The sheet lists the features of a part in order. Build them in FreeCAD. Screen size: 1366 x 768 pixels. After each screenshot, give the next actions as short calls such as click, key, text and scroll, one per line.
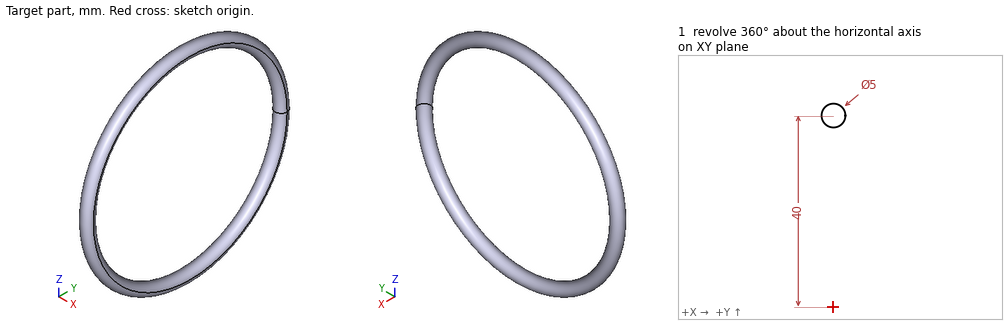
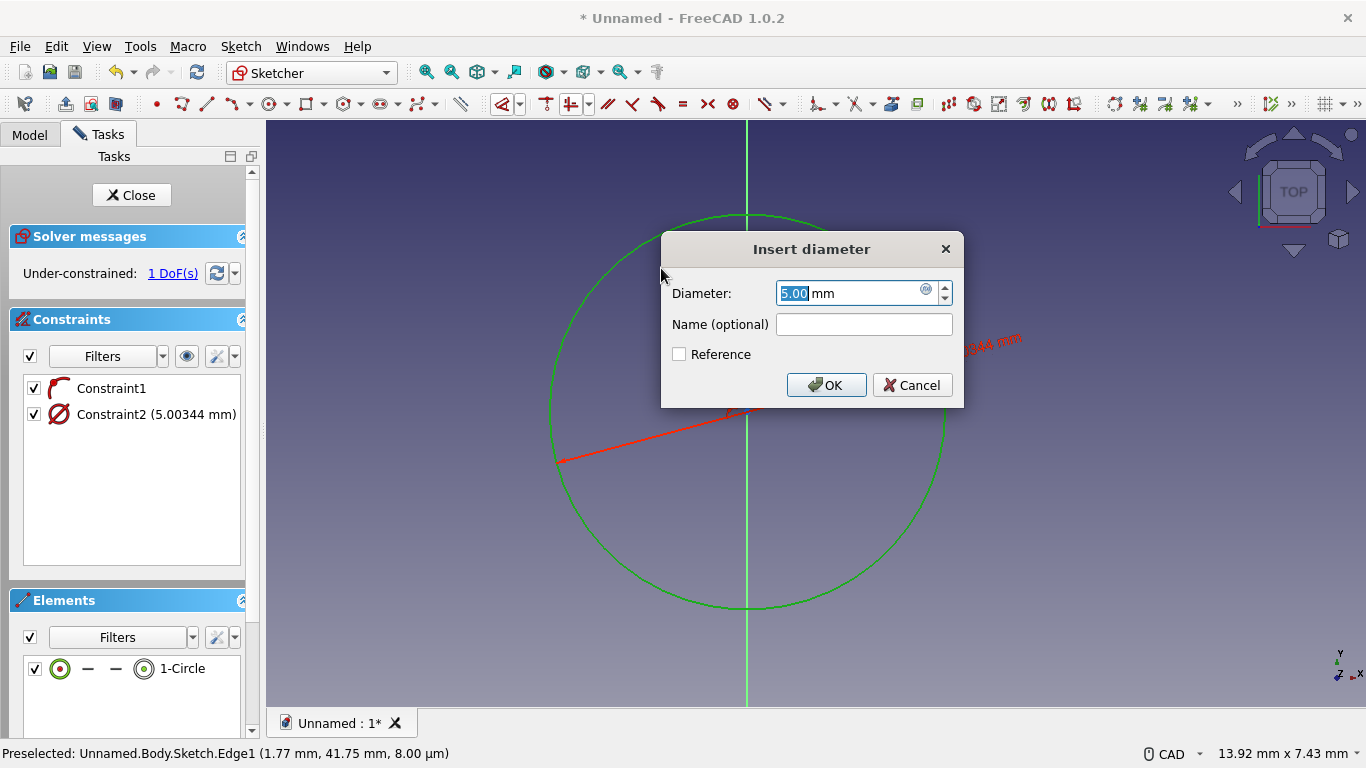
text(5)
key(Return)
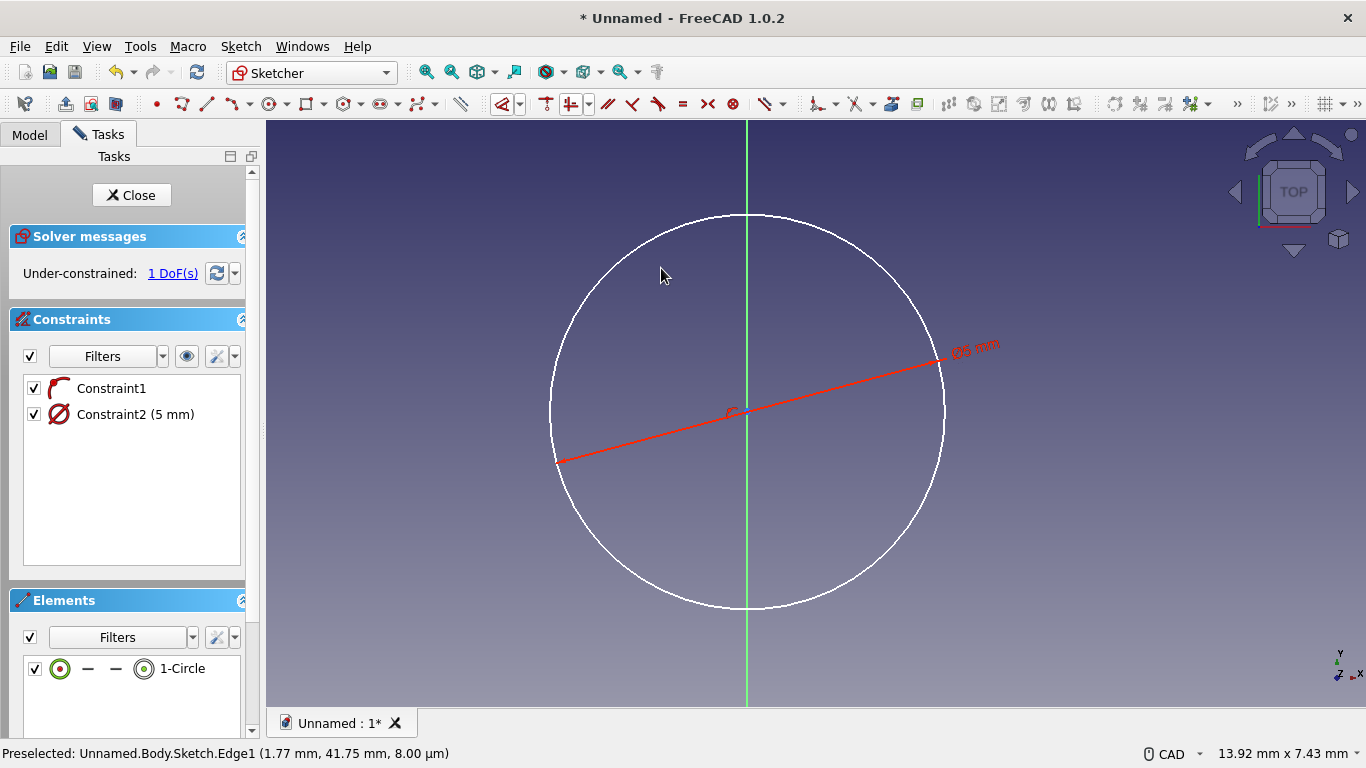
click(747, 412)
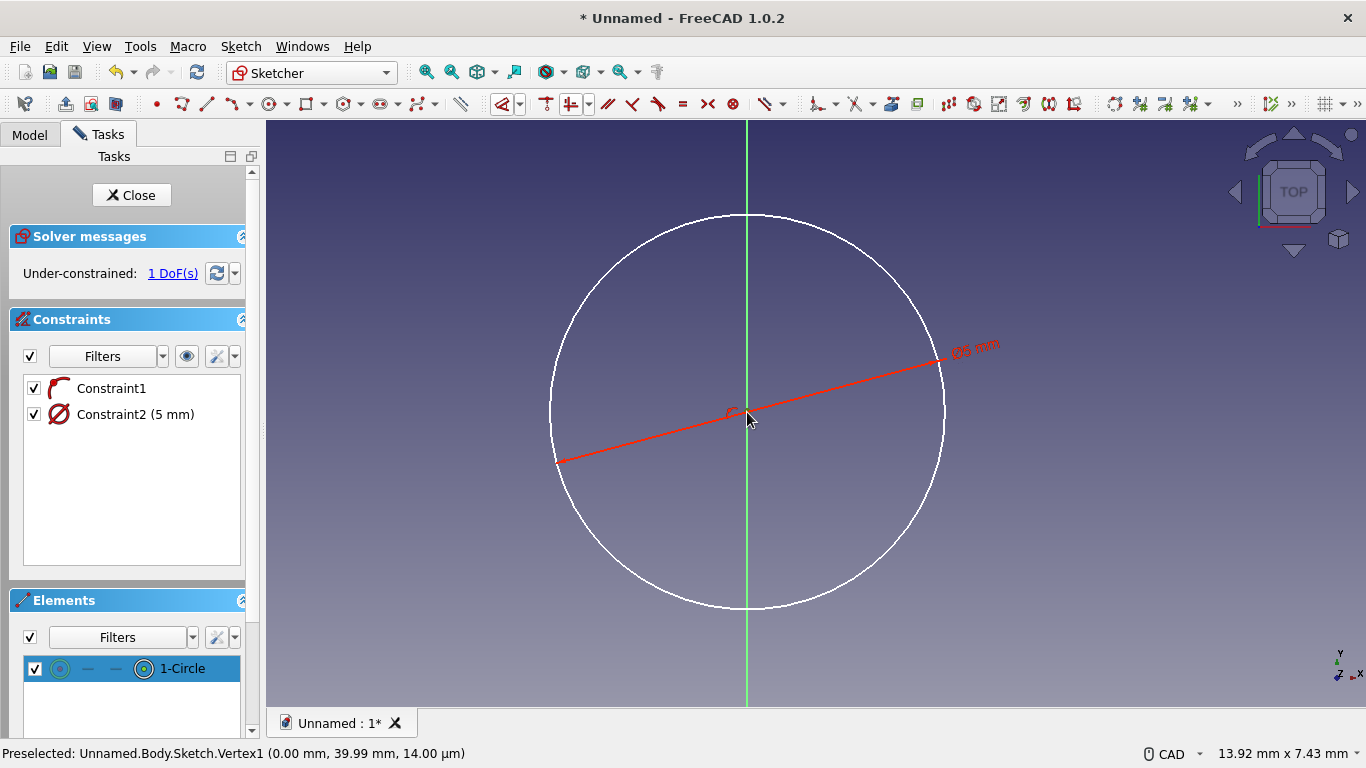
click(520, 104)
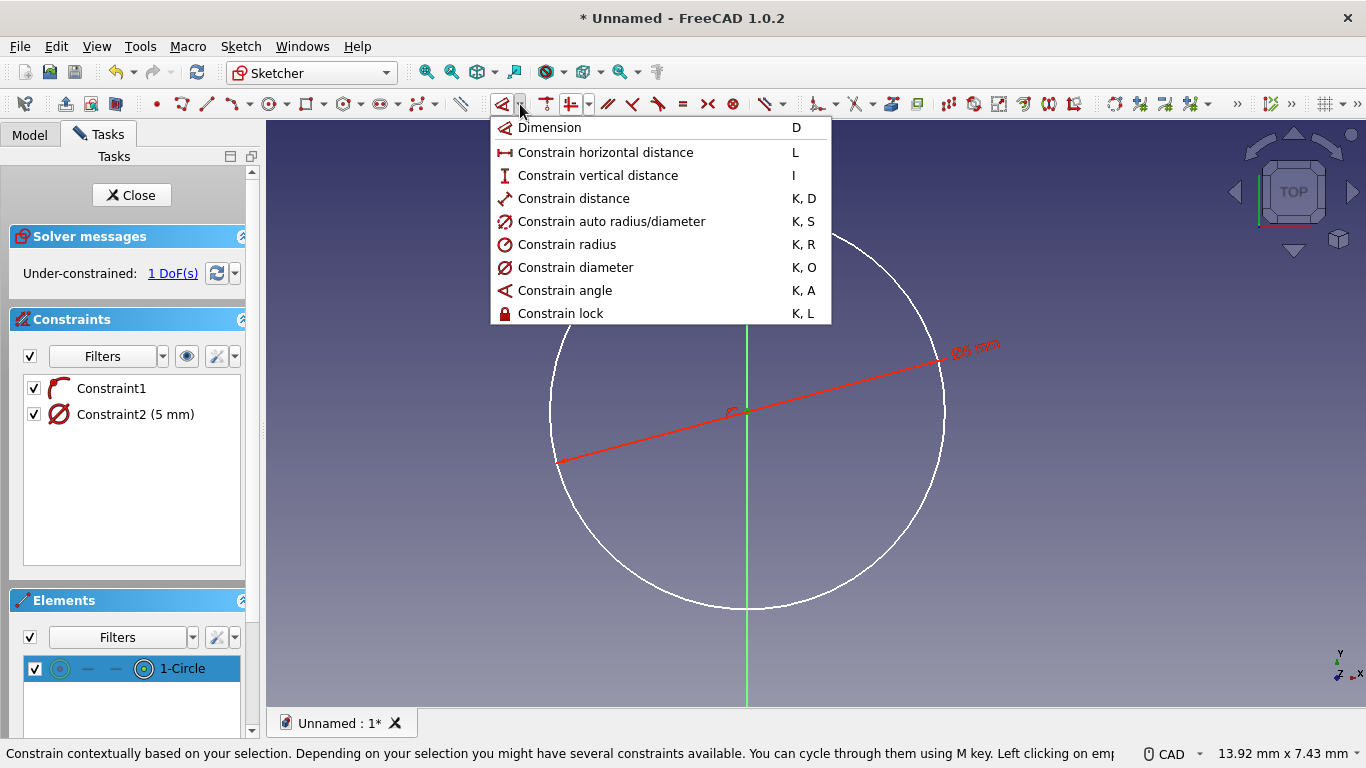
click(661, 176)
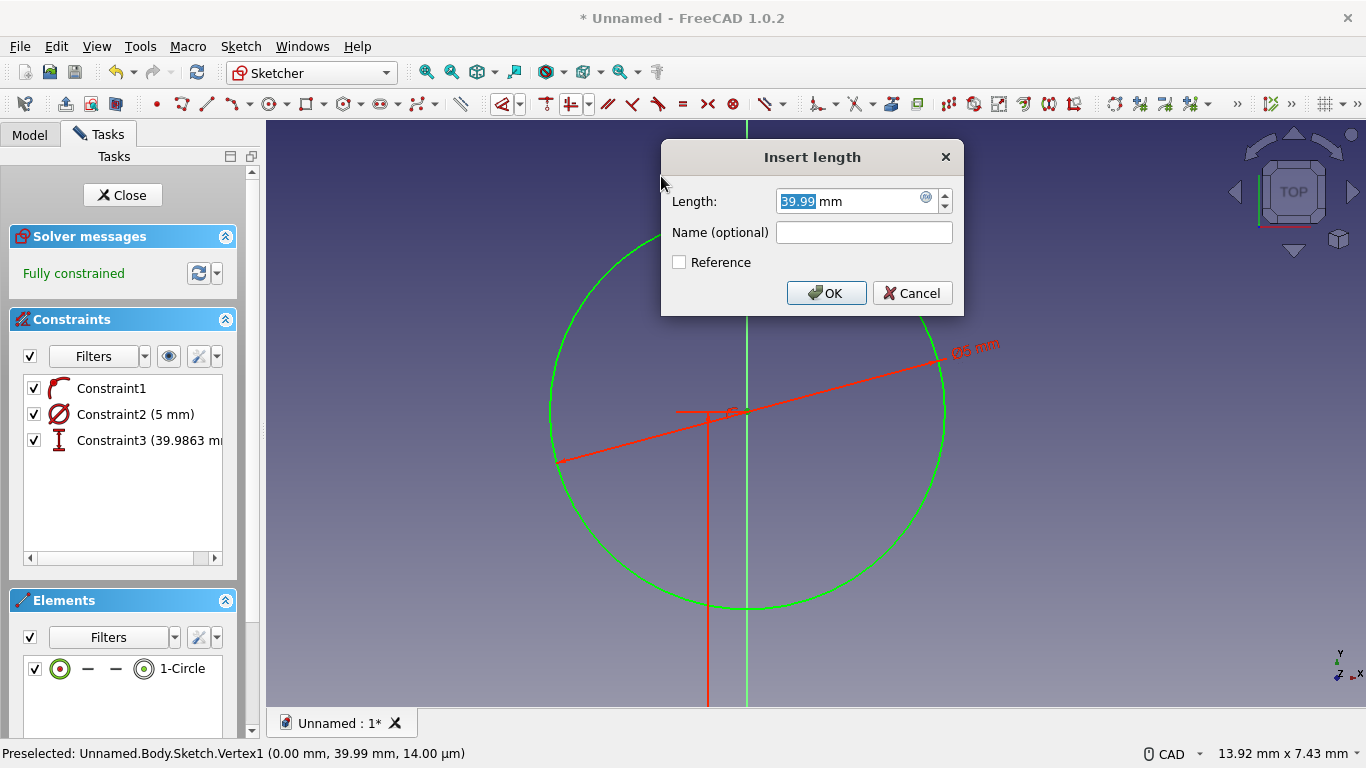
text(40)
key(Return)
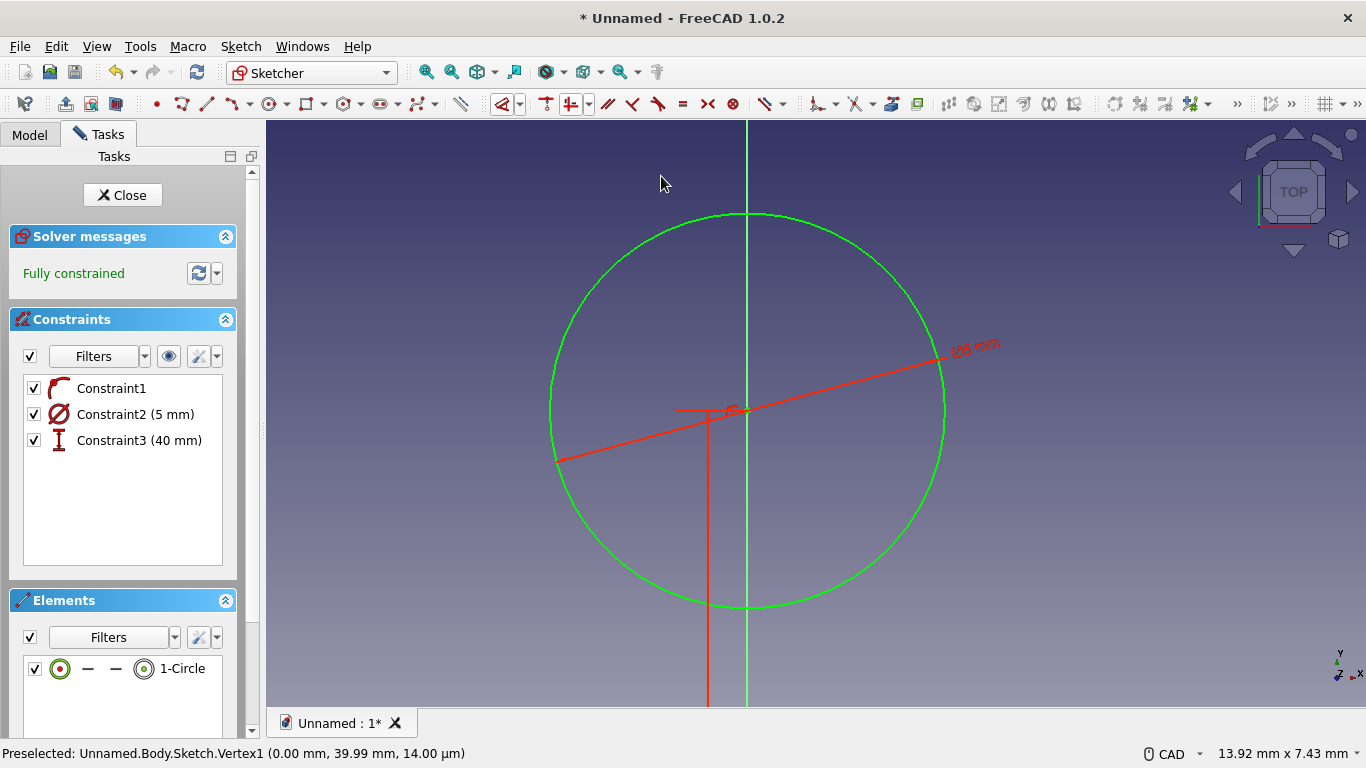
click(123, 195)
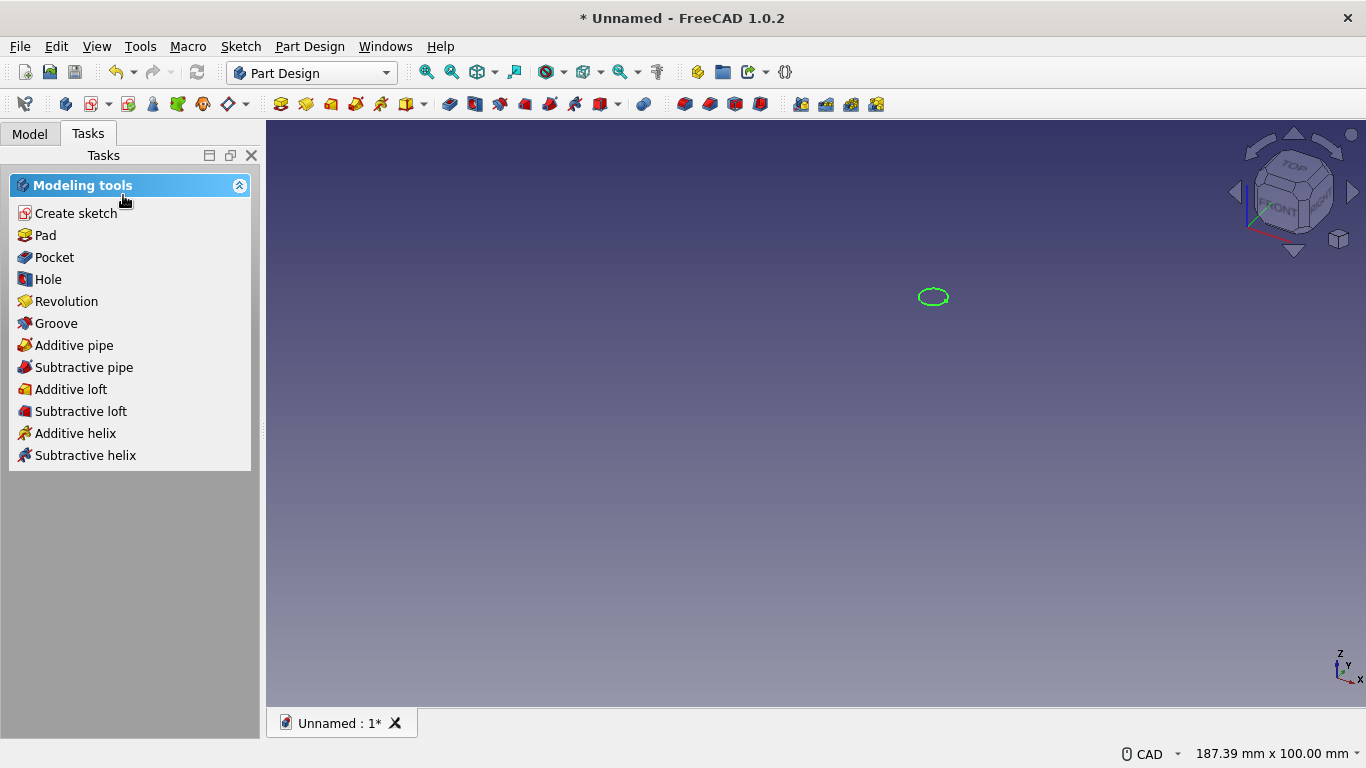
click(306, 104)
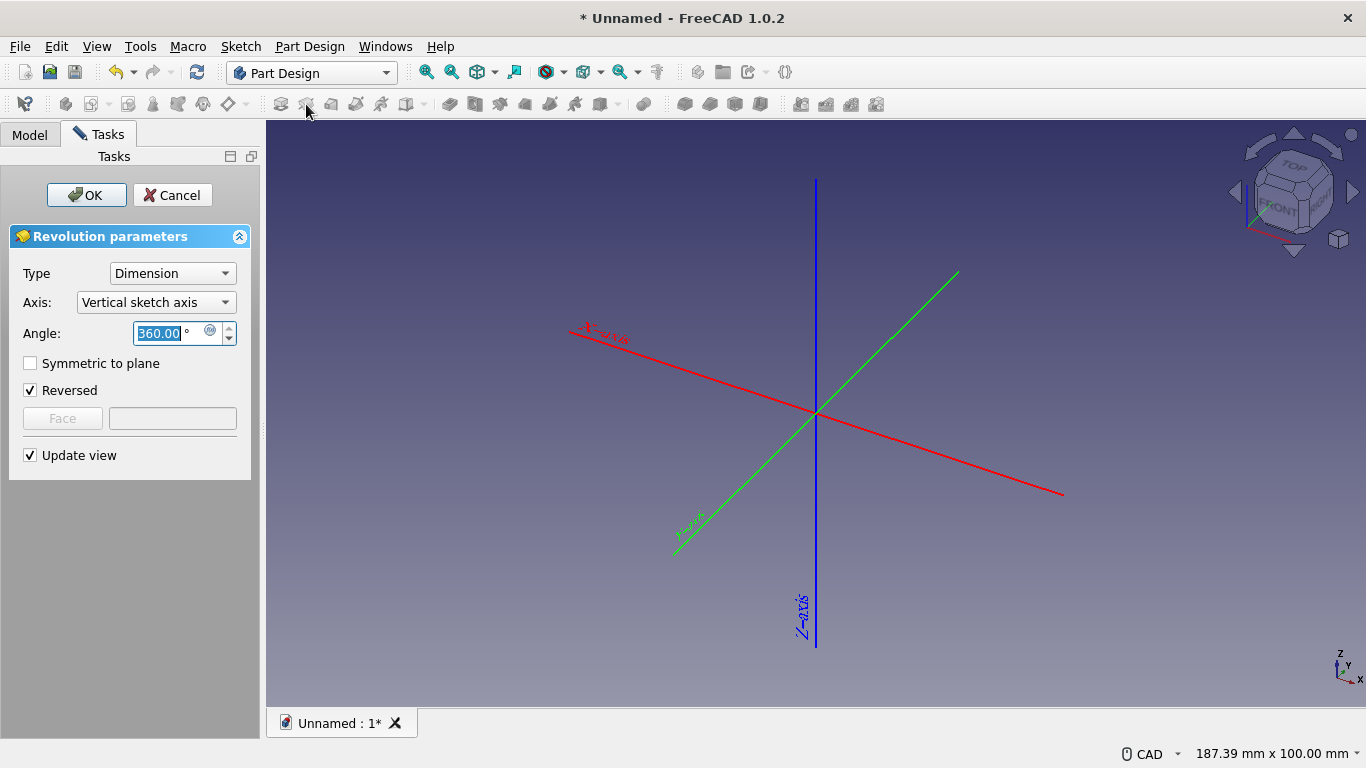
click(157, 302)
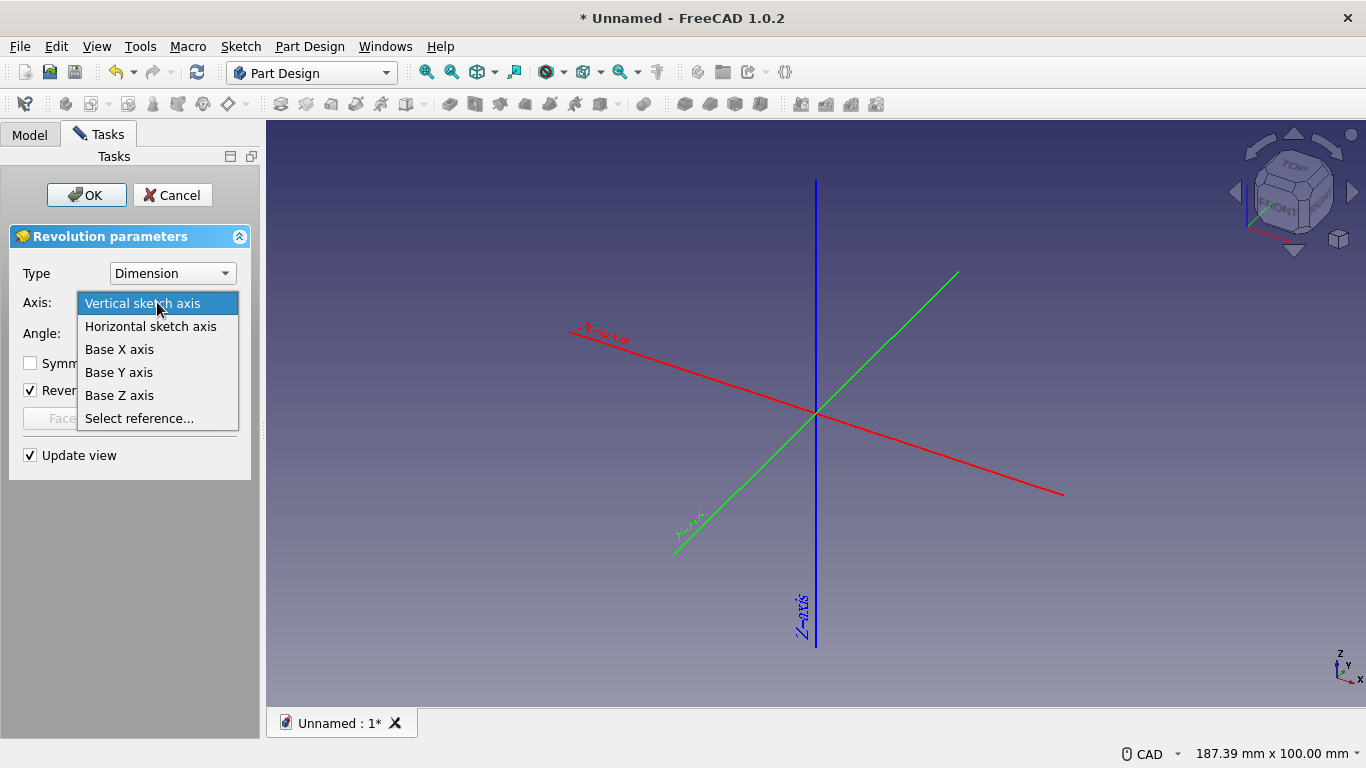
click(156, 326)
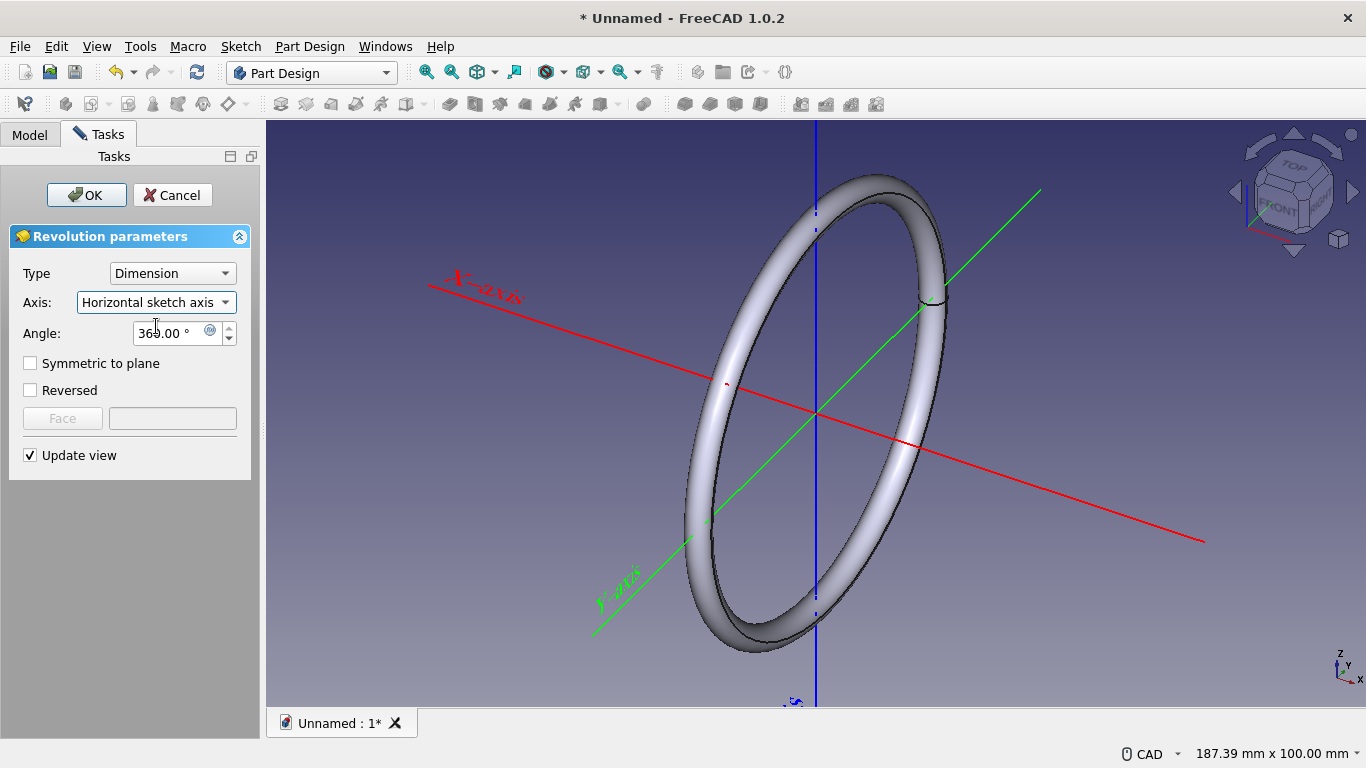
click(87, 195)